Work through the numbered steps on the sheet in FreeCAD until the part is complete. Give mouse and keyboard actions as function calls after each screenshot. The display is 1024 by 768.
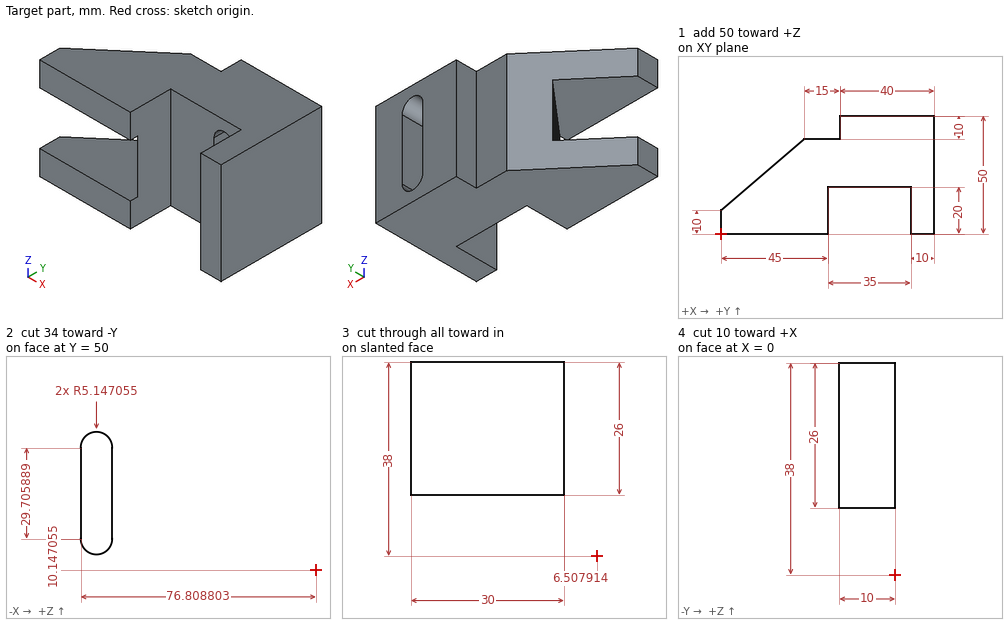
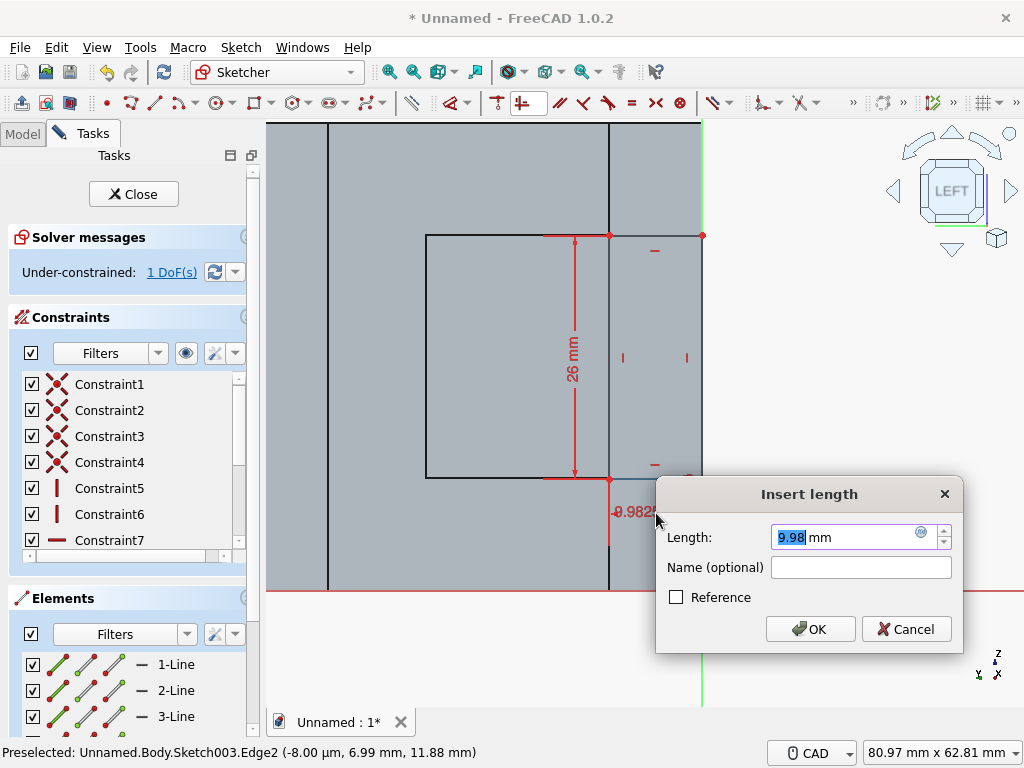
text(10)
key(Return)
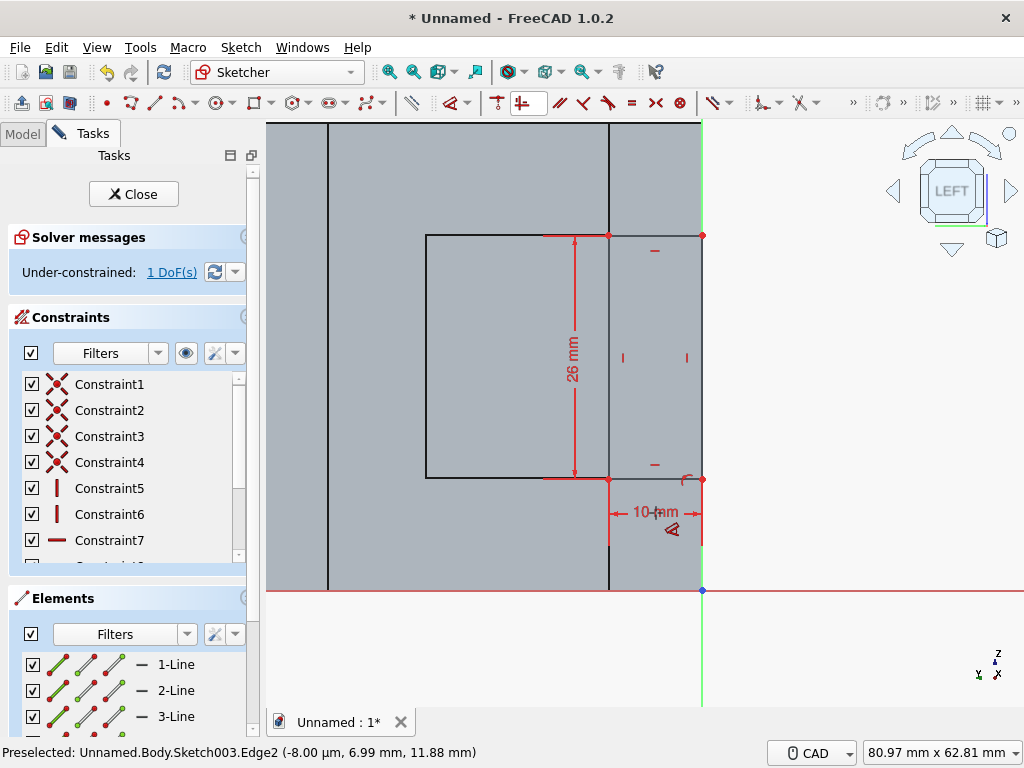
click(609, 236)
click(736, 413)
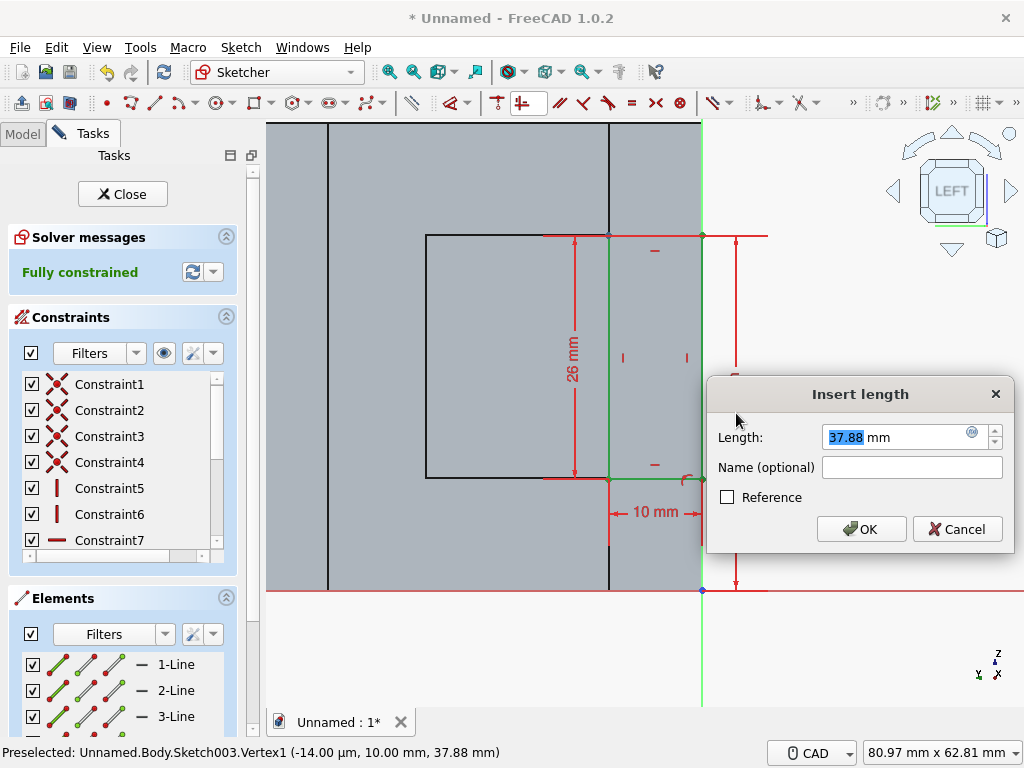
text(38)
key(Return)
key(Escape)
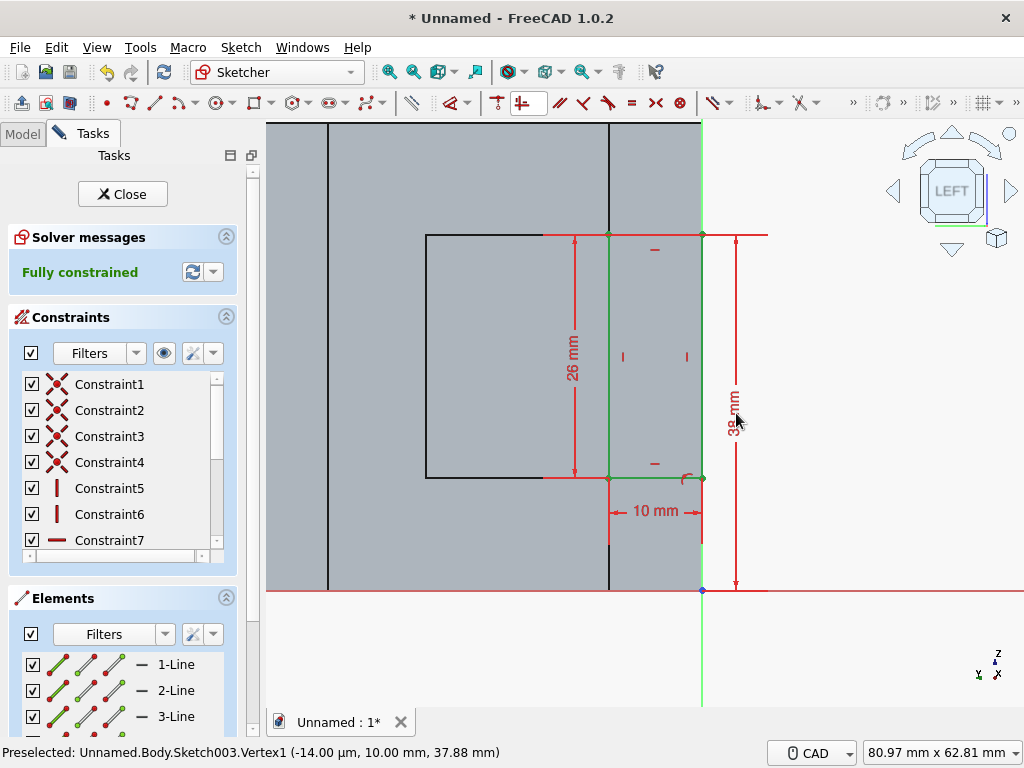
click(123, 194)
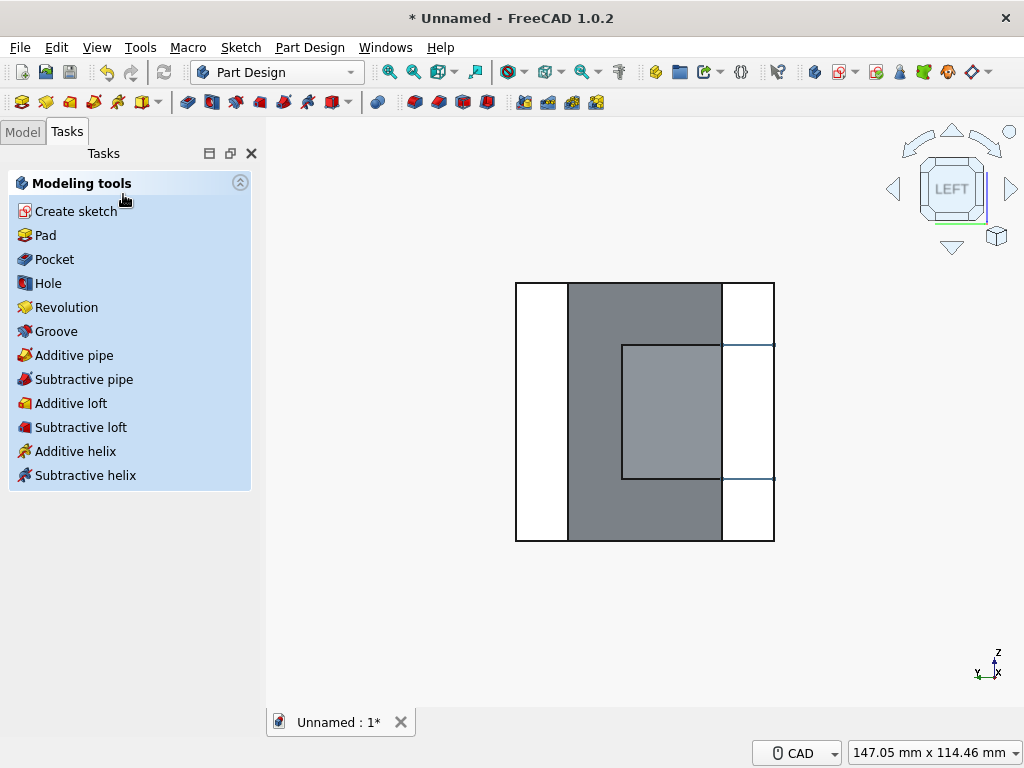
click(188, 102)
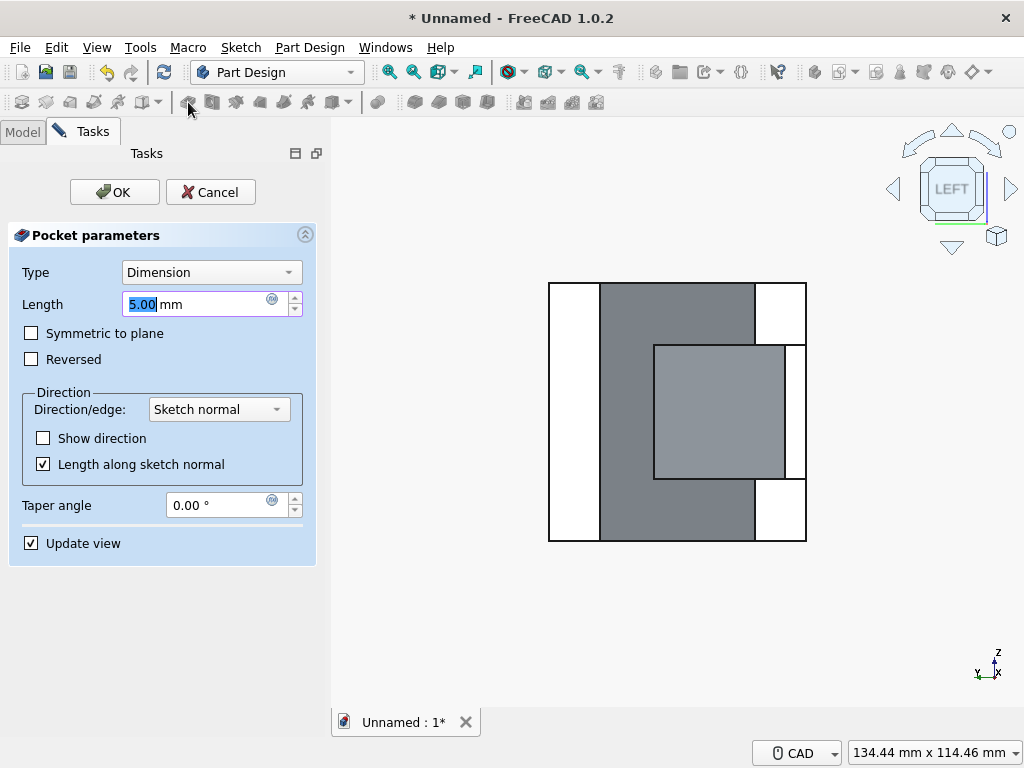
text(10)
key(Tab)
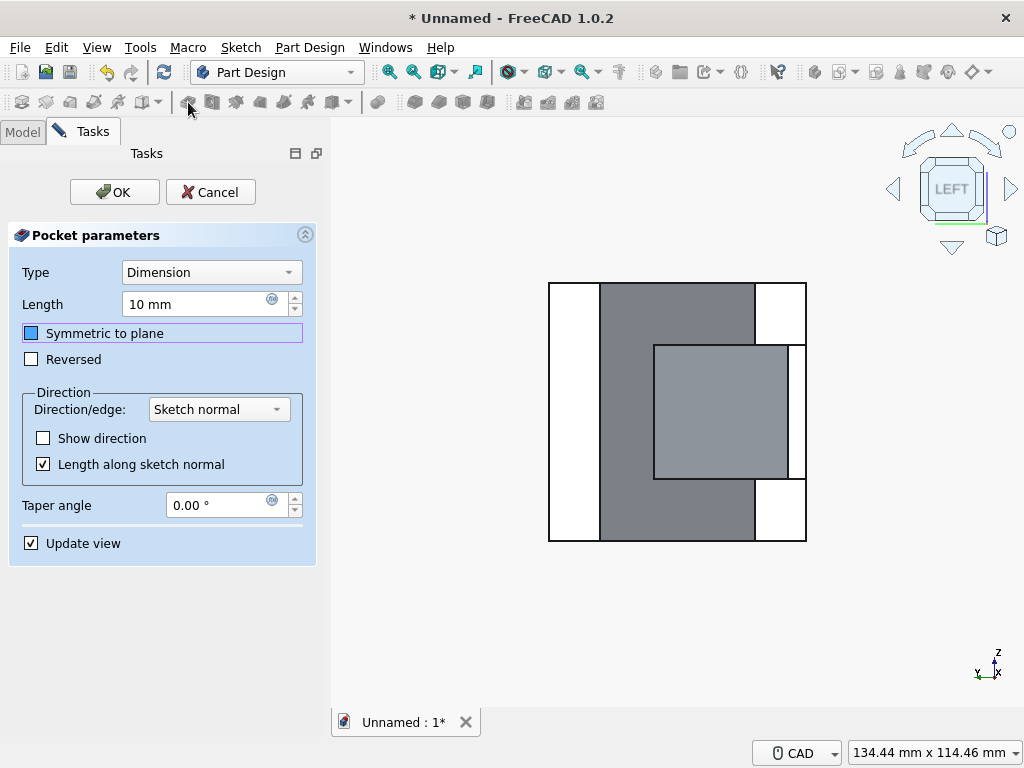
click(115, 192)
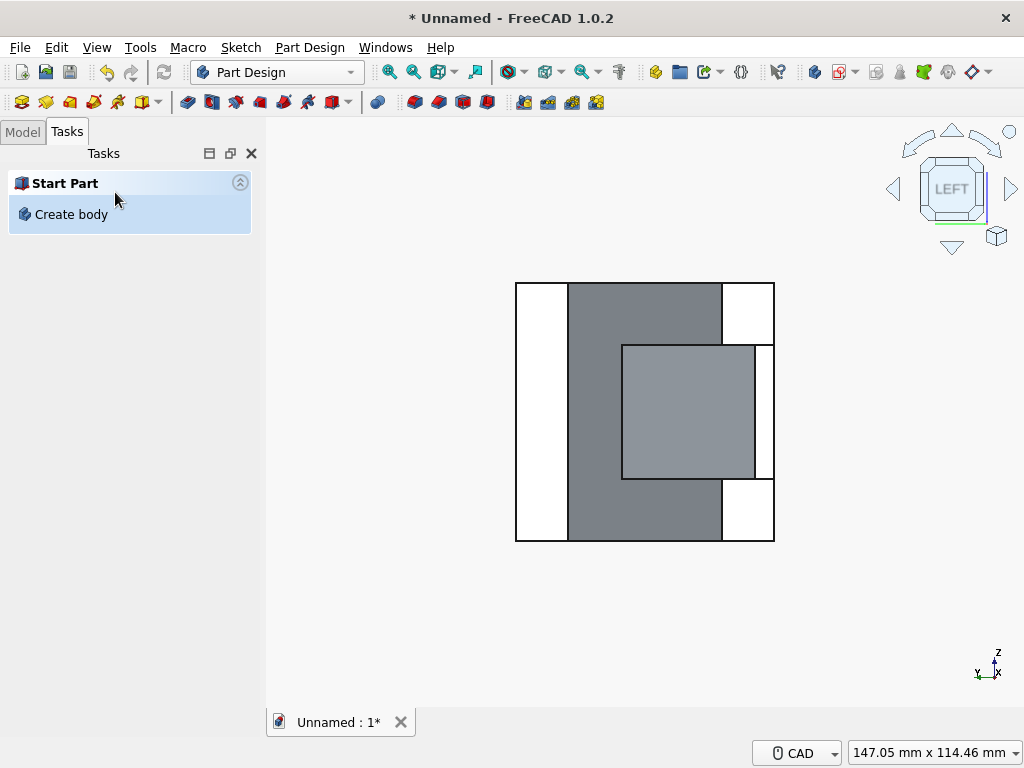
key(0)